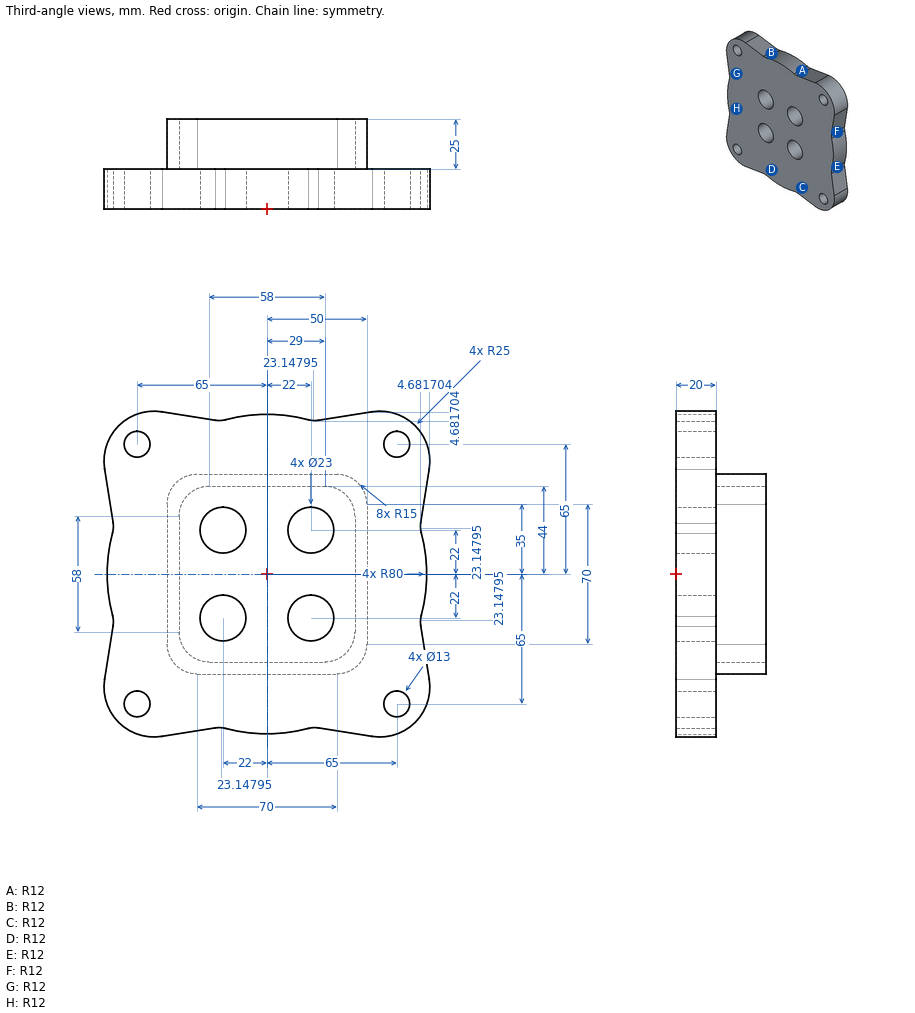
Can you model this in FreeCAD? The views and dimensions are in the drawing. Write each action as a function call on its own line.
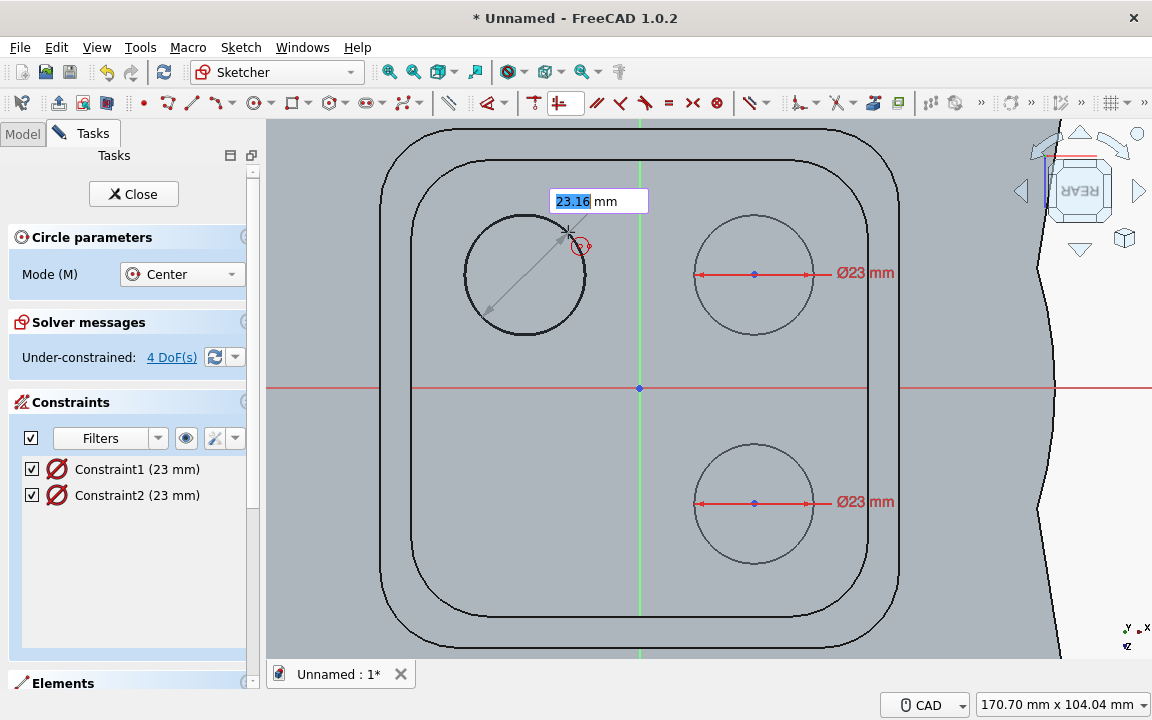
text(23)
key(Return)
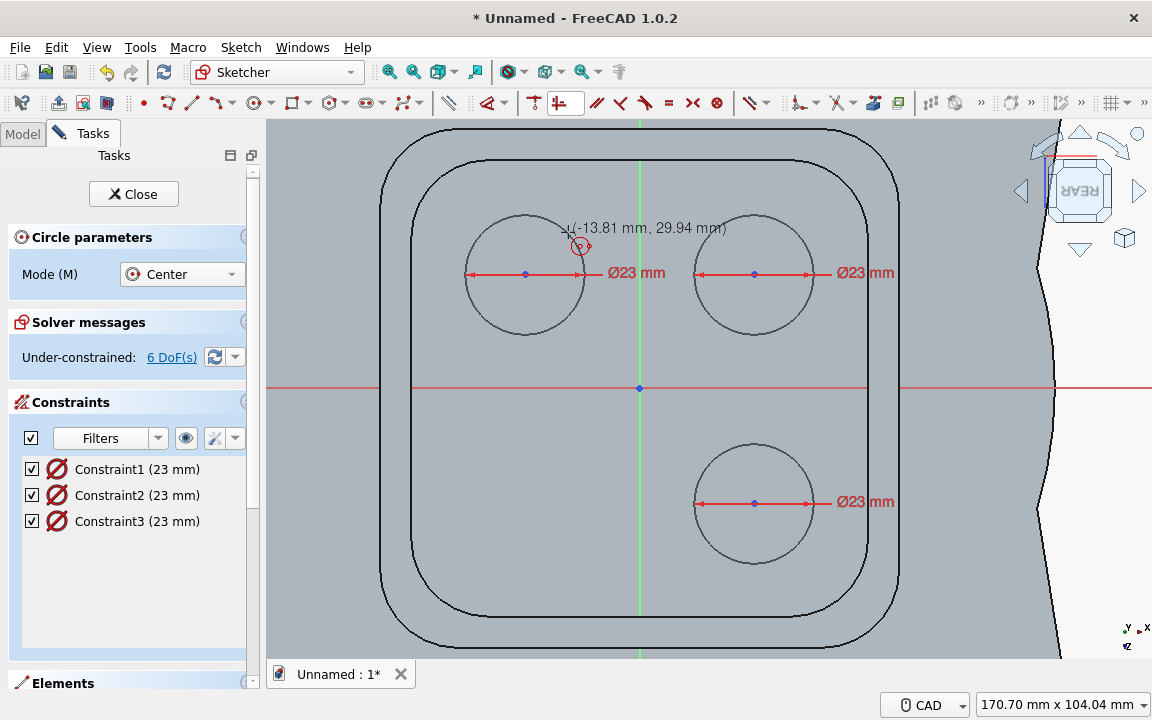
click(525, 503)
move(568, 460)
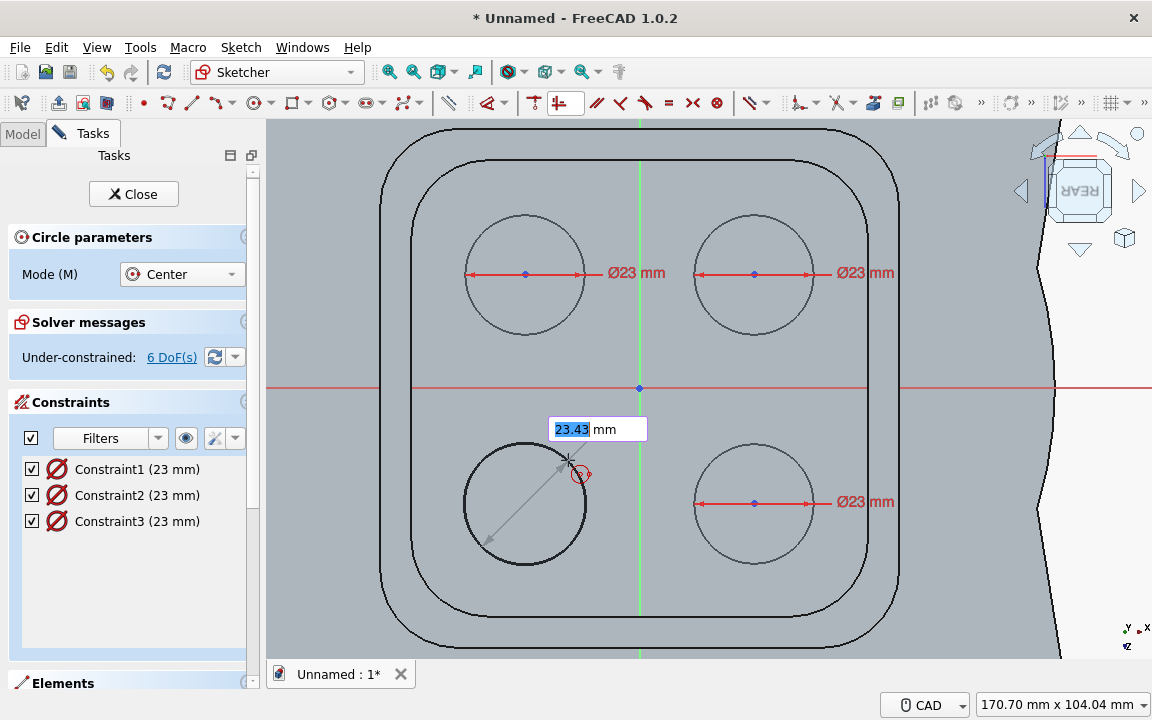
text(23)
key(Return)
key(Escape)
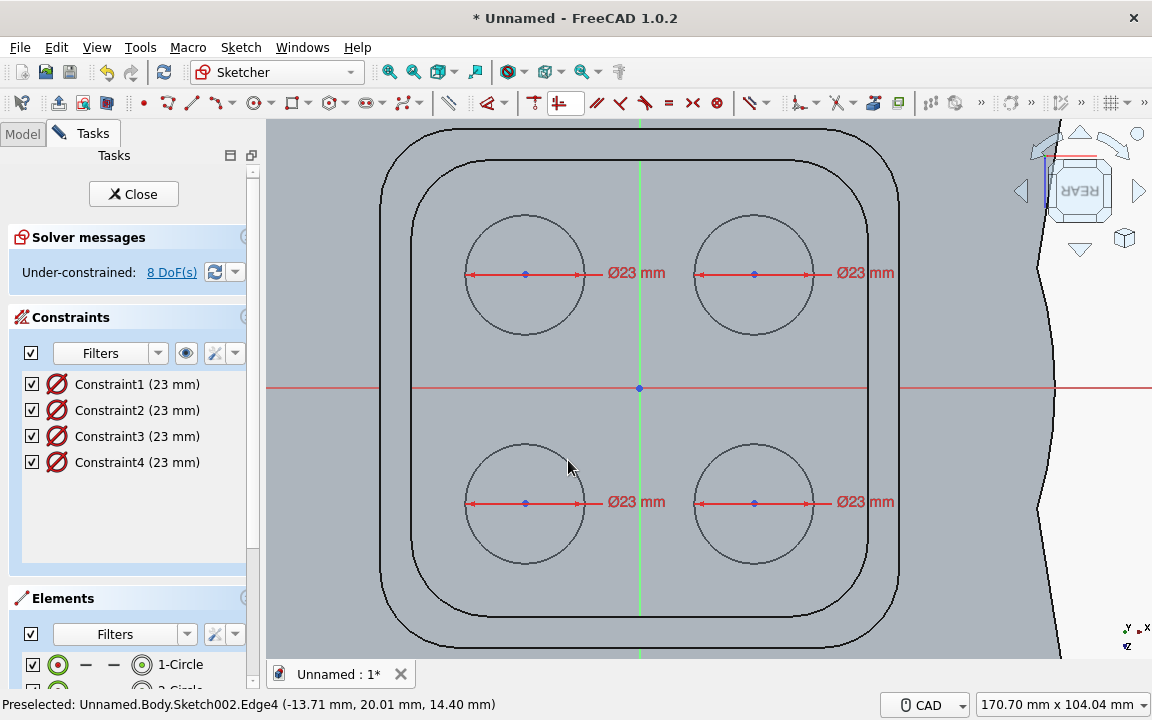
click(754, 504)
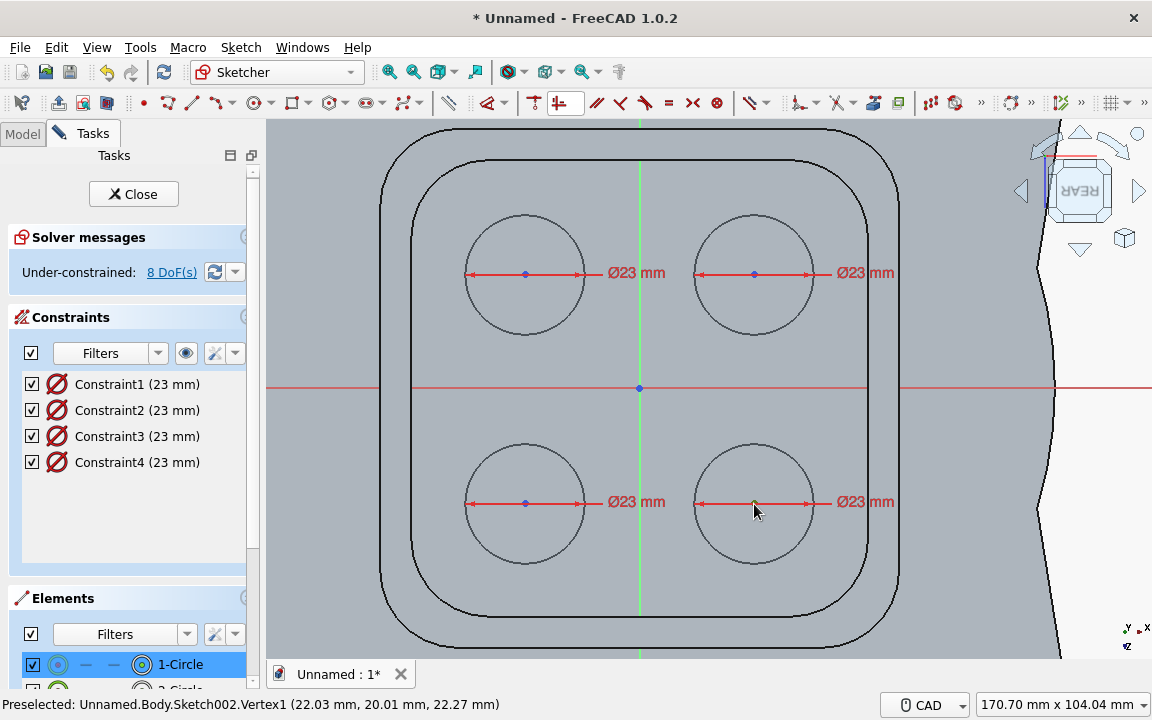
click(754, 275)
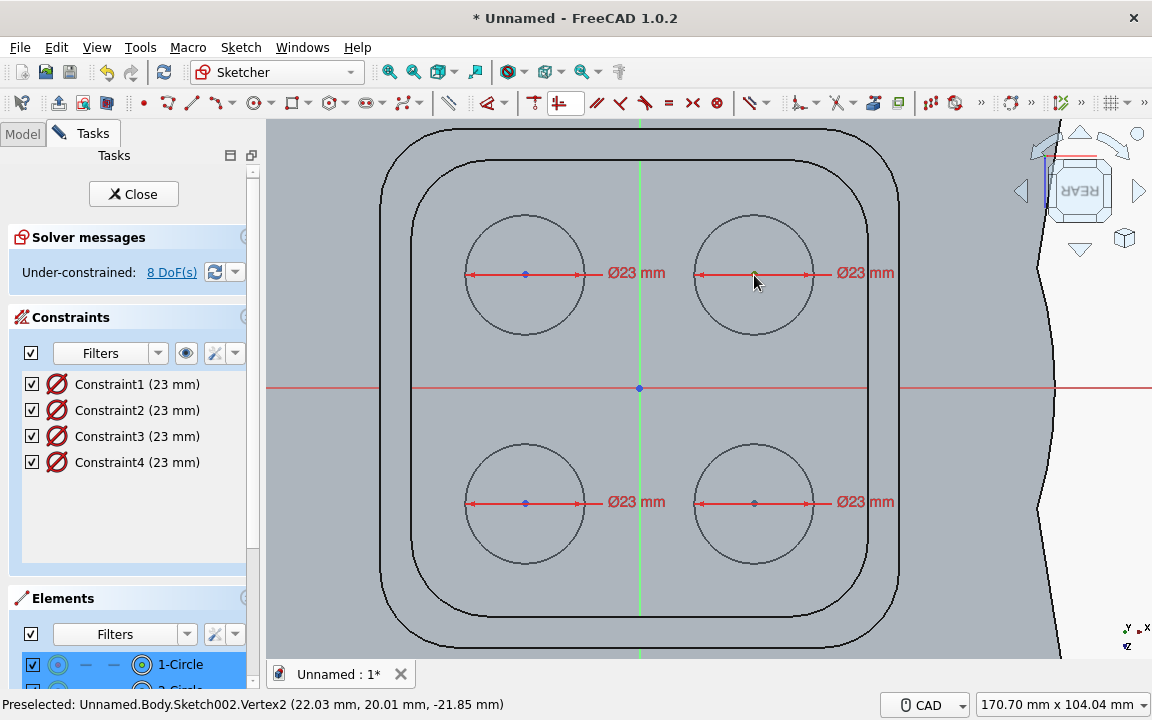
click(578, 104)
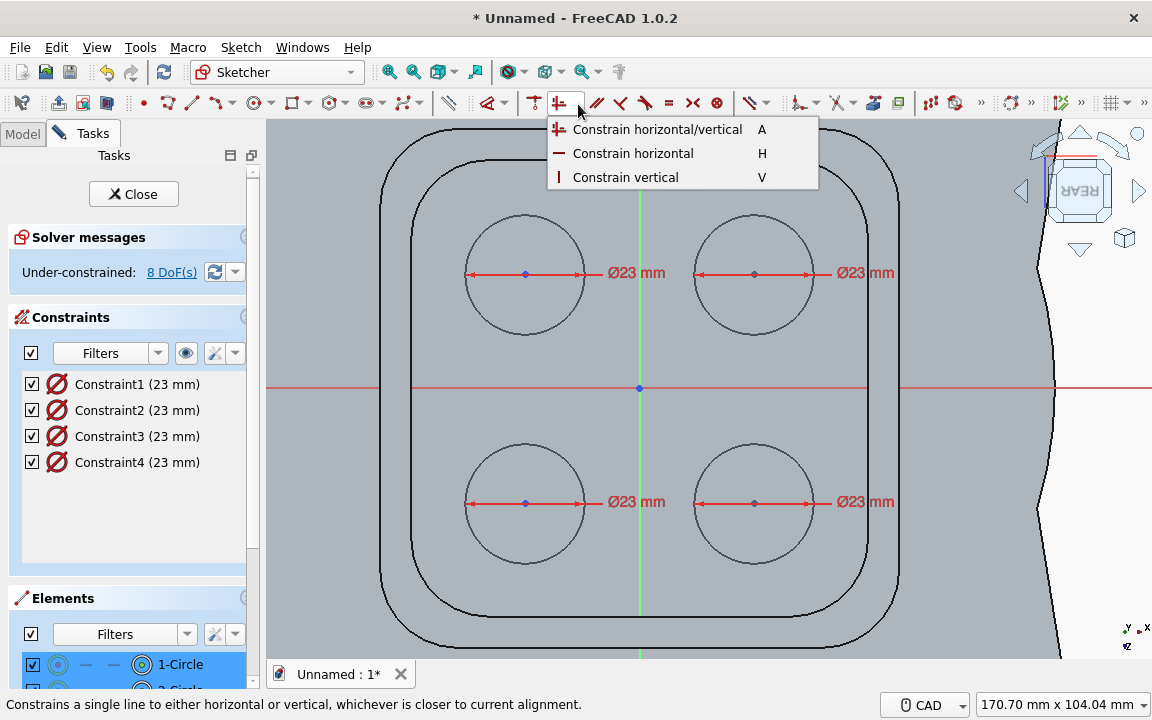
click(683, 177)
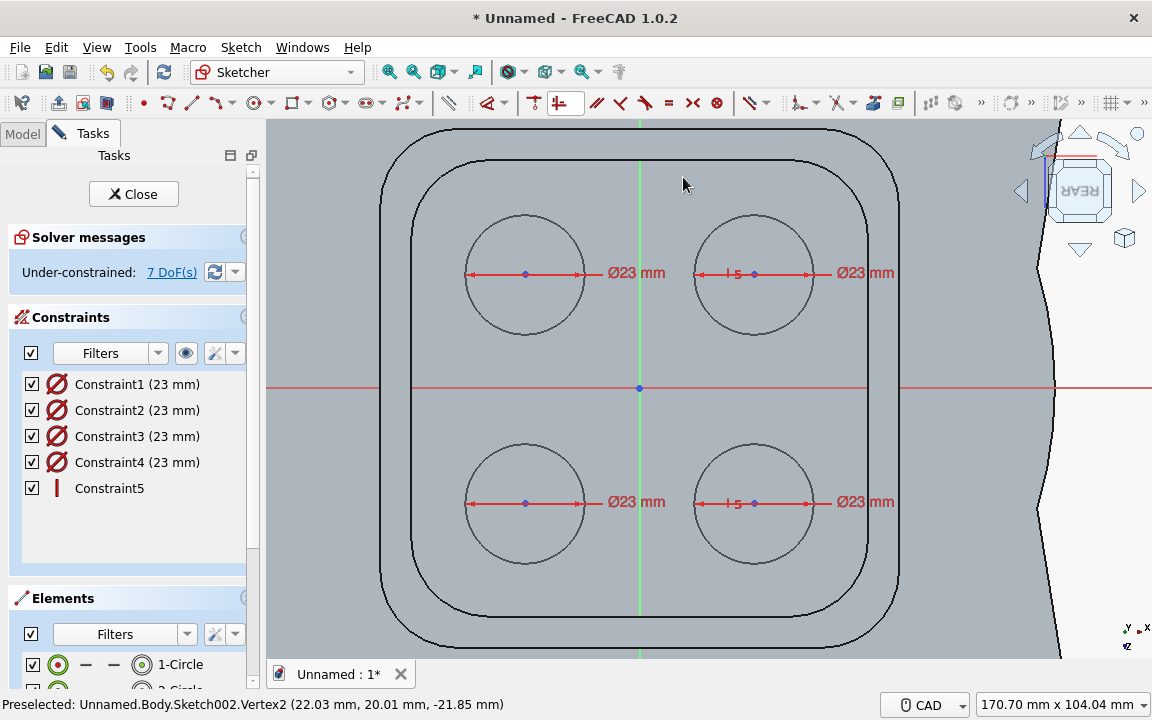
click(754, 275)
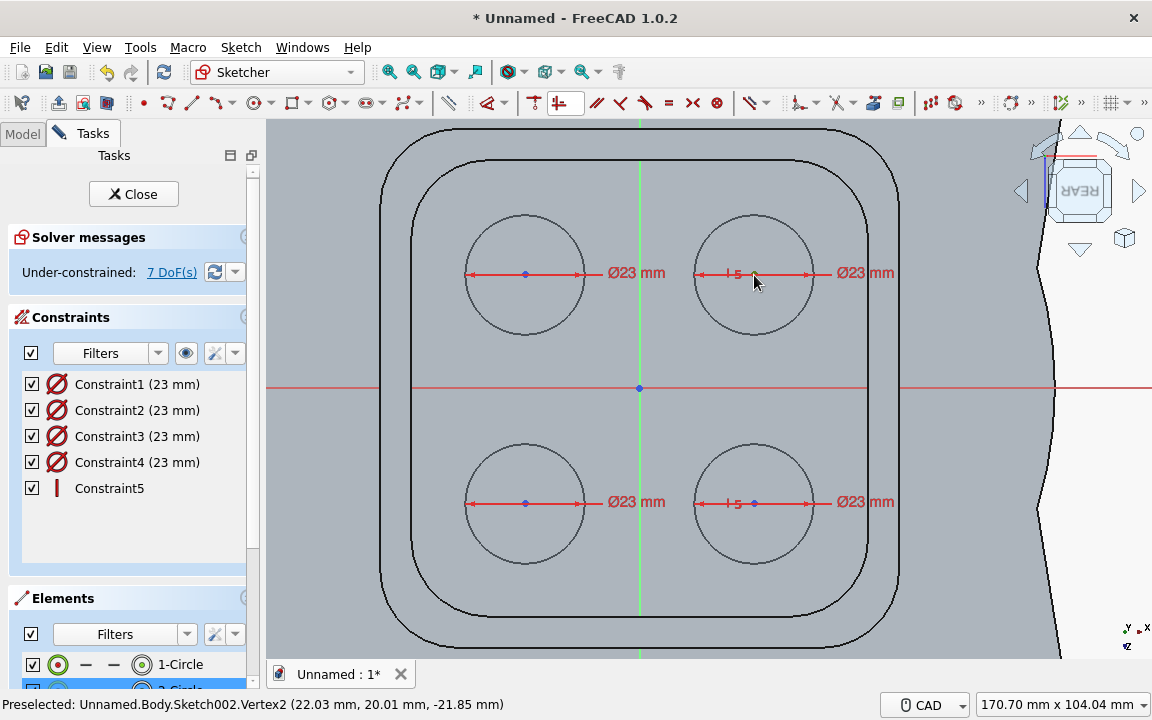
click(525, 275)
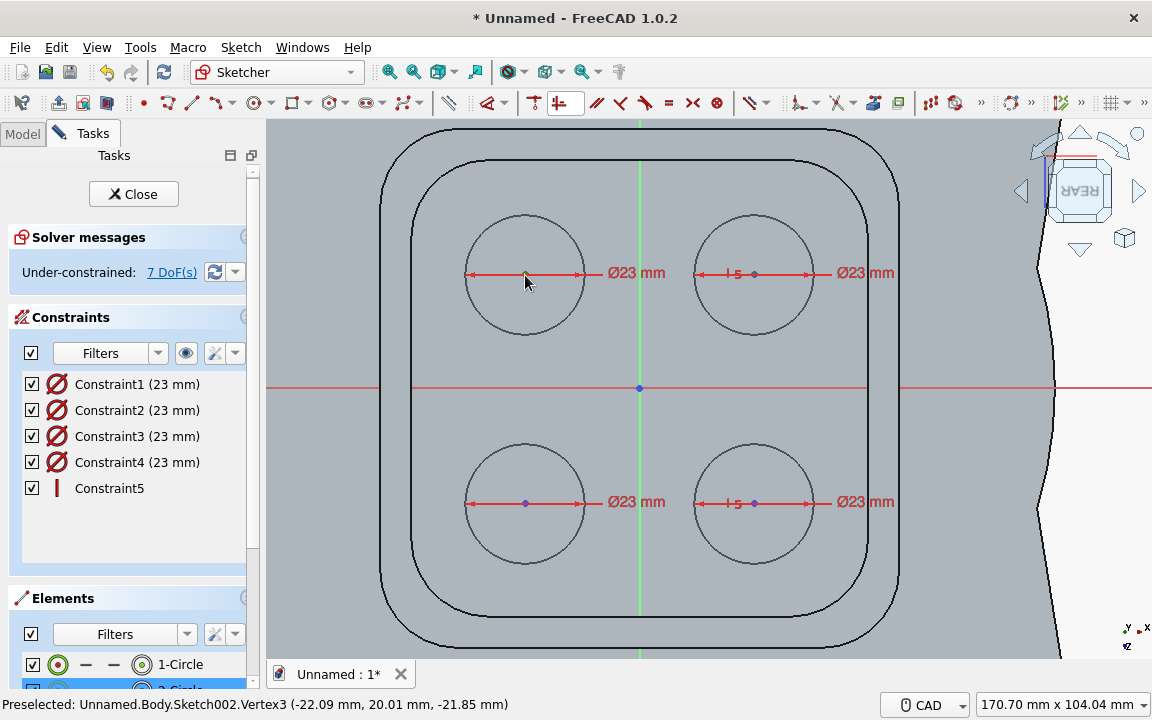
click(578, 104)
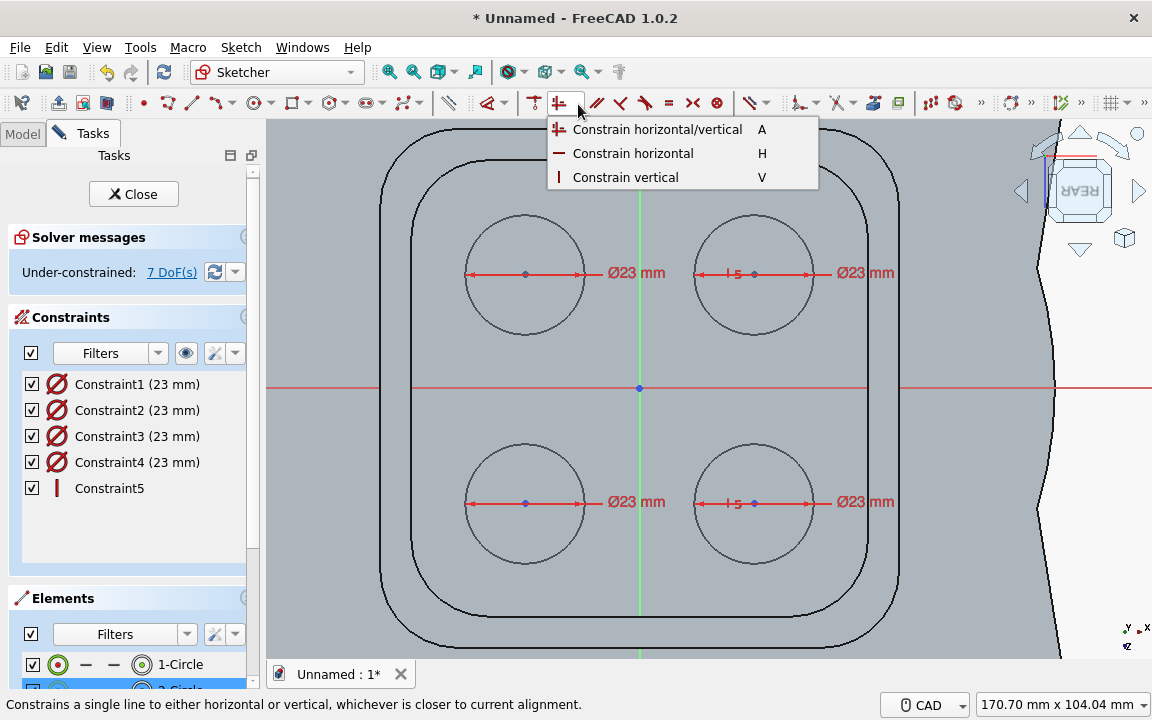
click(683, 153)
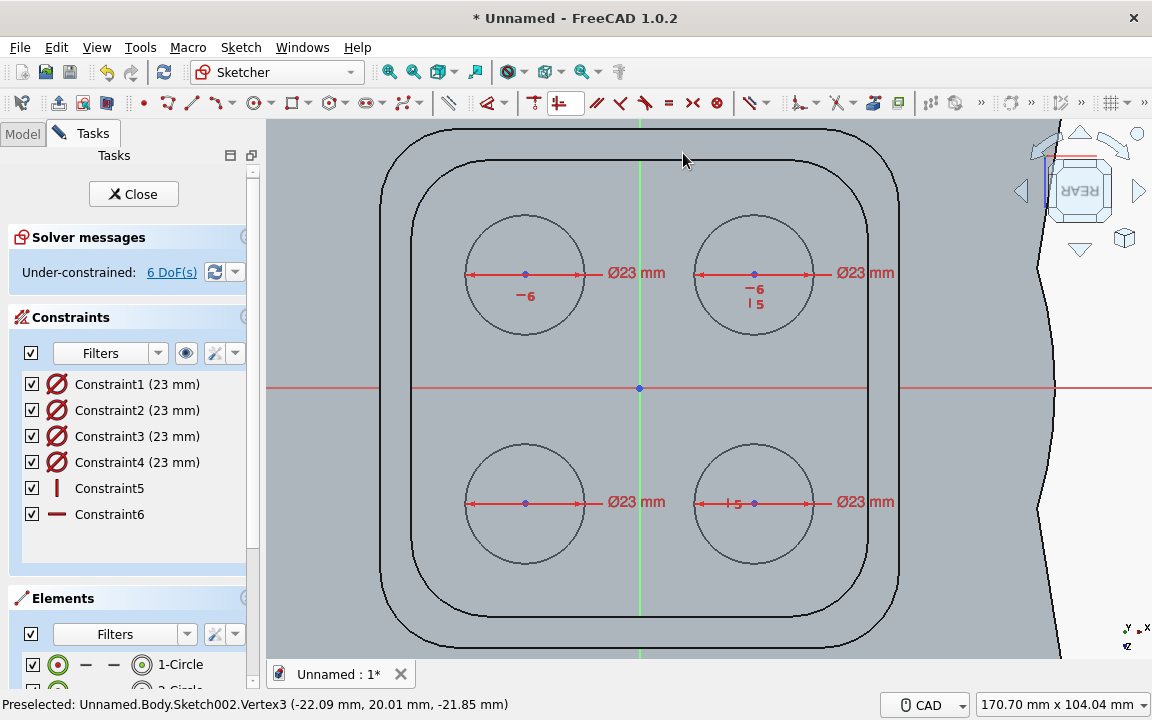
click(525, 275)